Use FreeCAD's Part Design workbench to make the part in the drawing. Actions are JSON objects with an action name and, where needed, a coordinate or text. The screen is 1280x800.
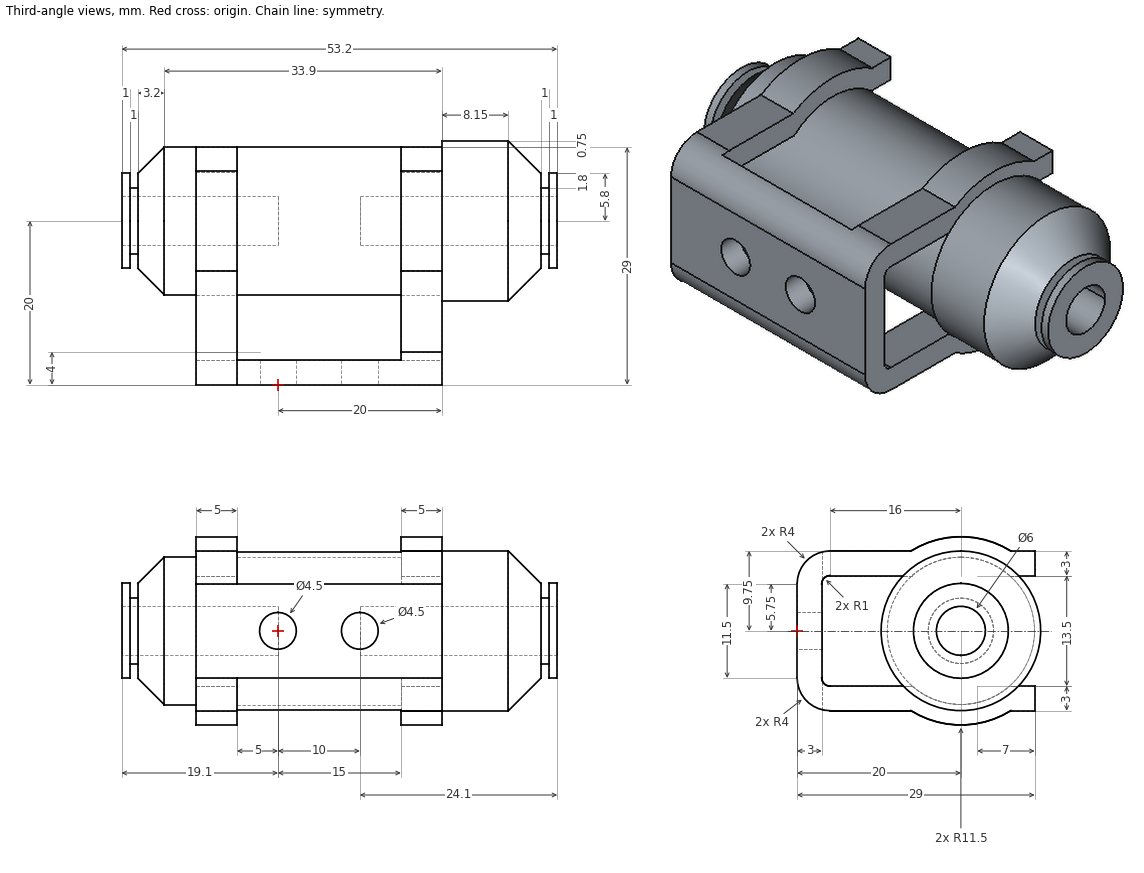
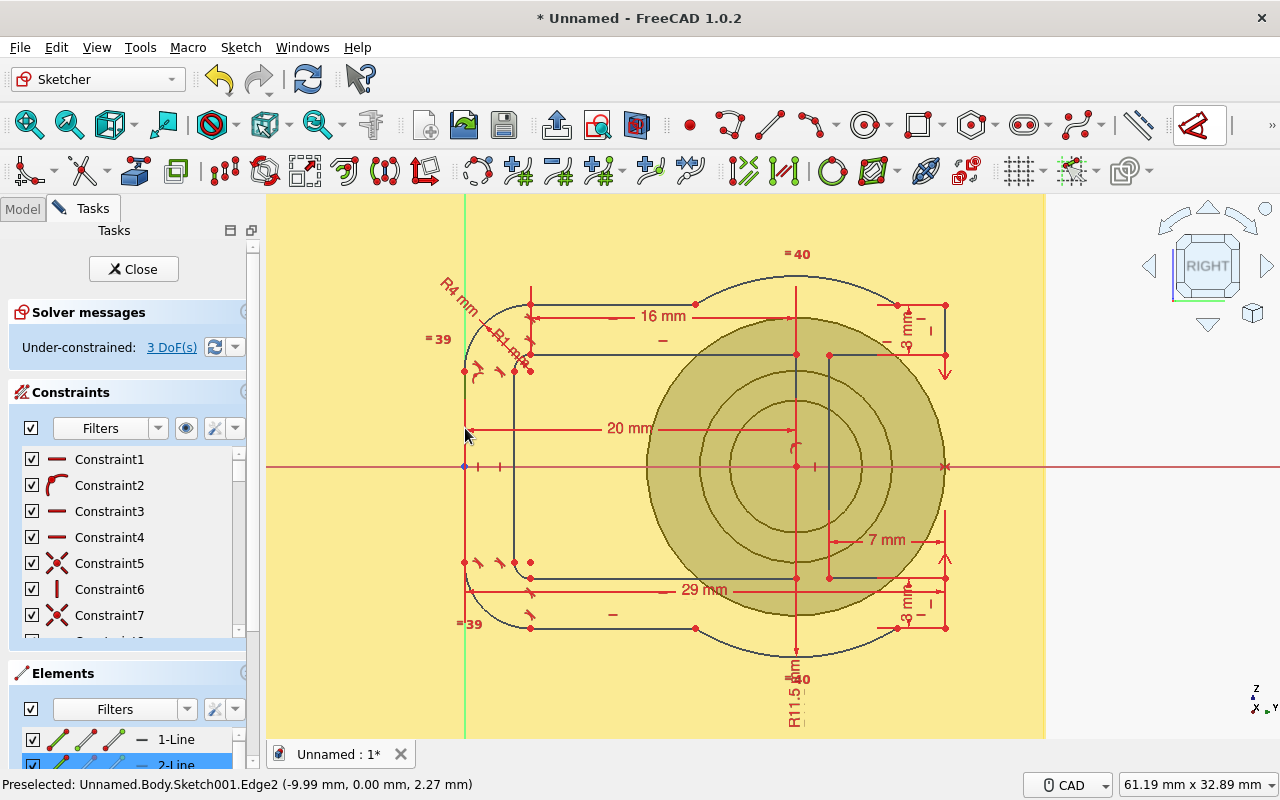
{"action": "left_click", "coordinate": [1220, 126]}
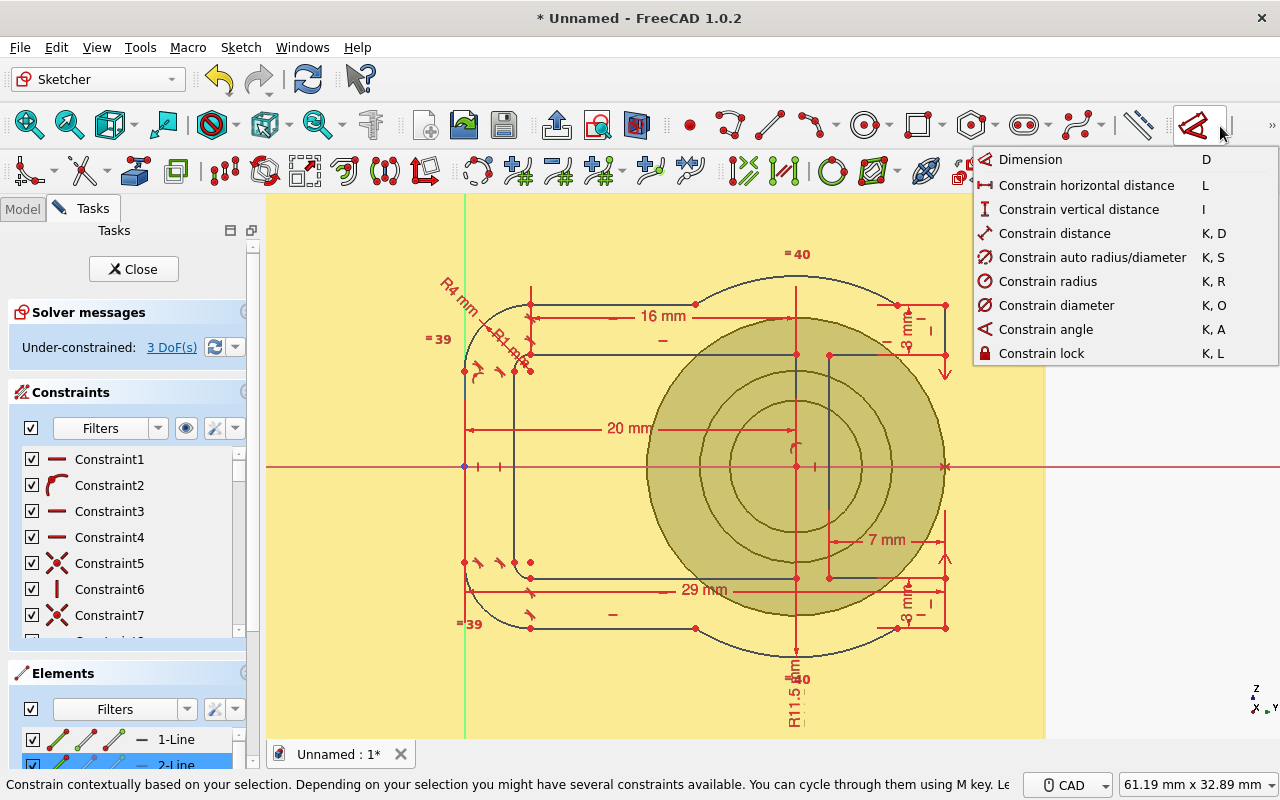
{"action": "left_click", "coordinate": [1126, 209]}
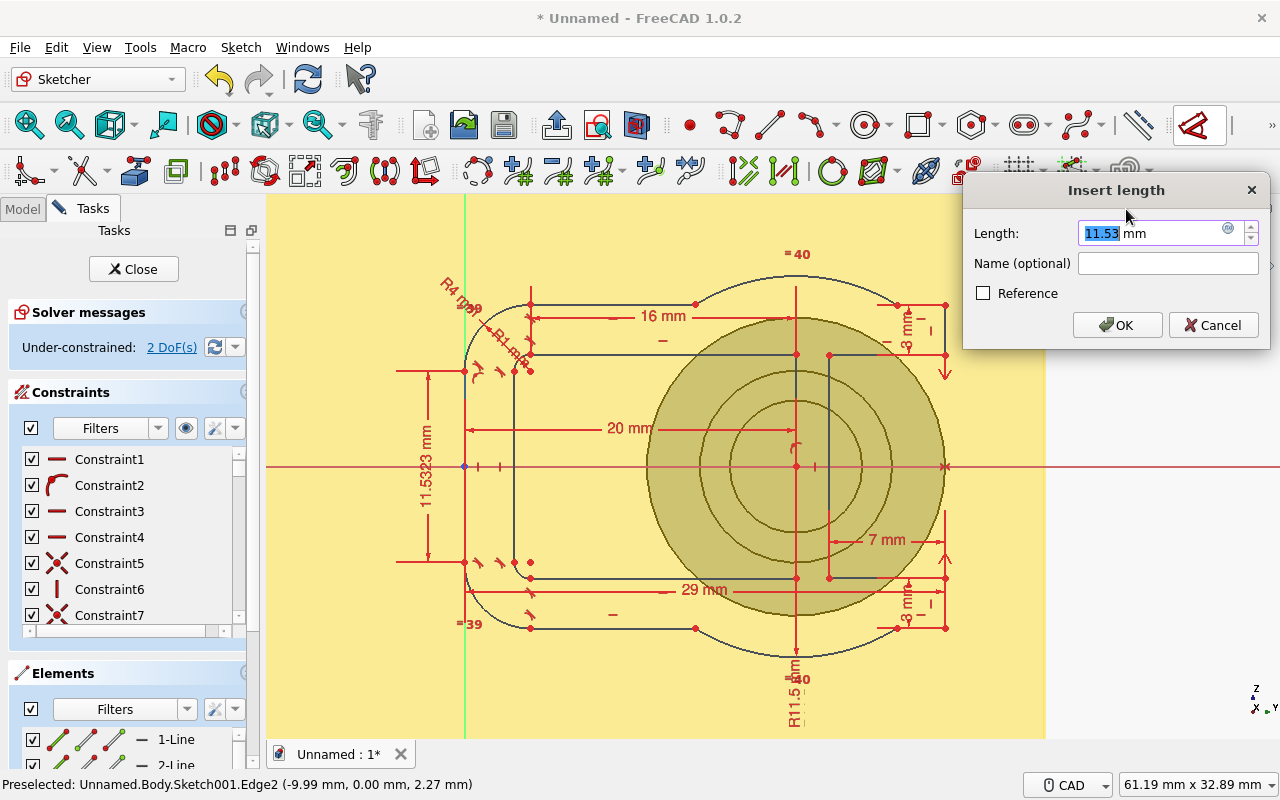
{"action": "type", "text": "11.5"}
{"action": "key", "text": "Return"}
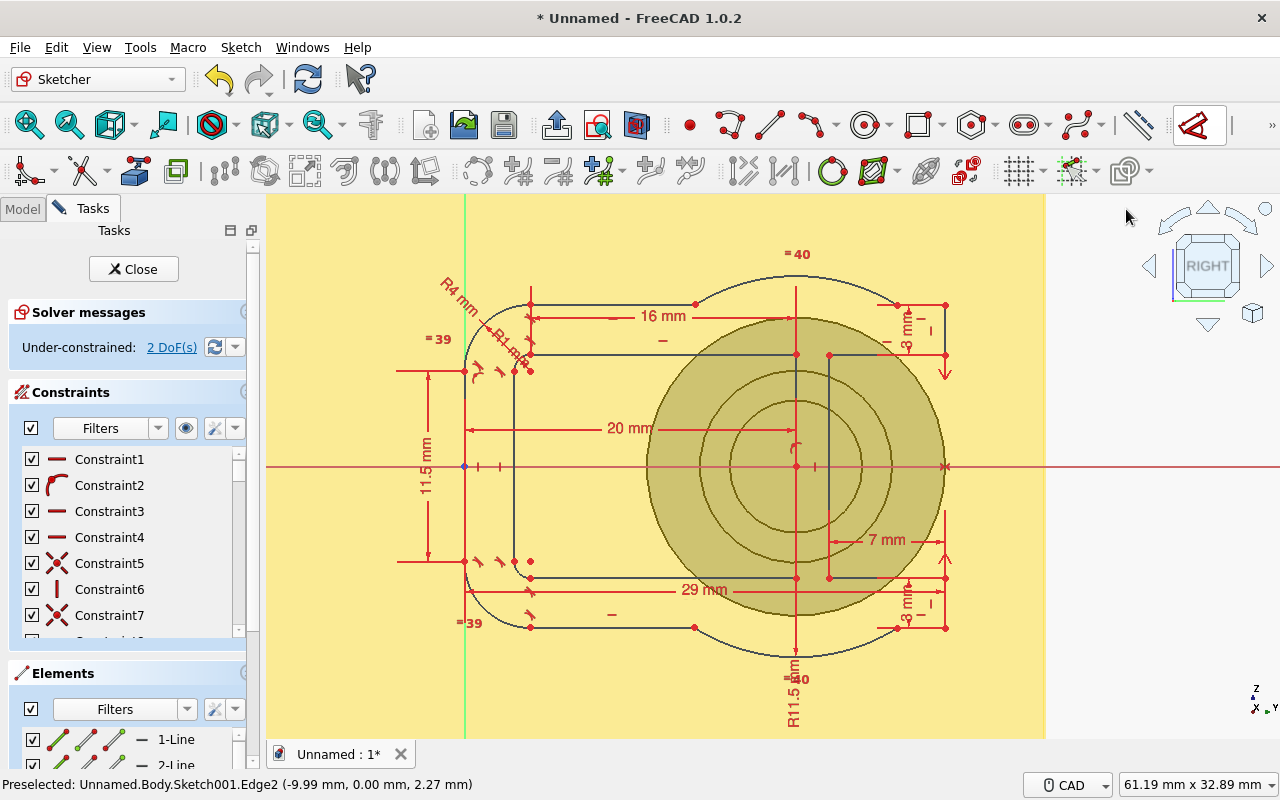
{"action": "left_click", "coordinate": [829, 511]}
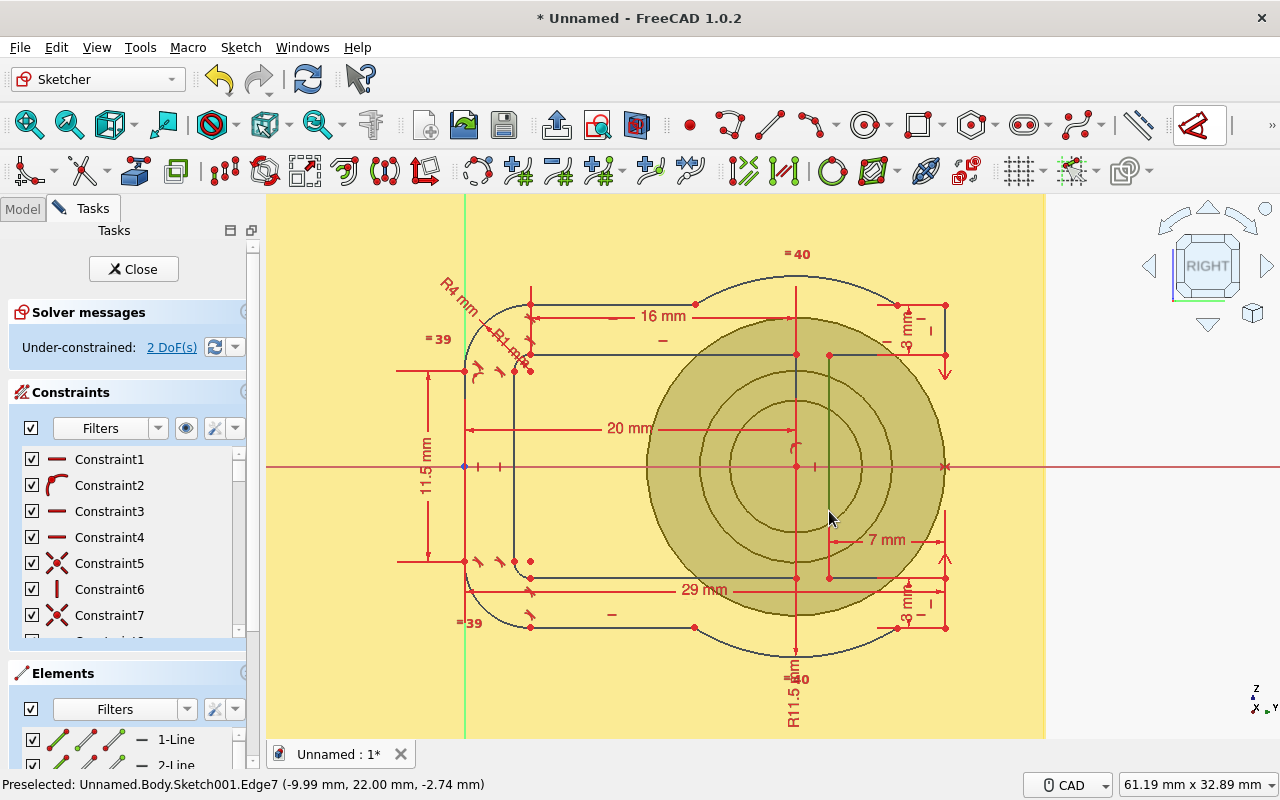
{"action": "key", "text": "i"}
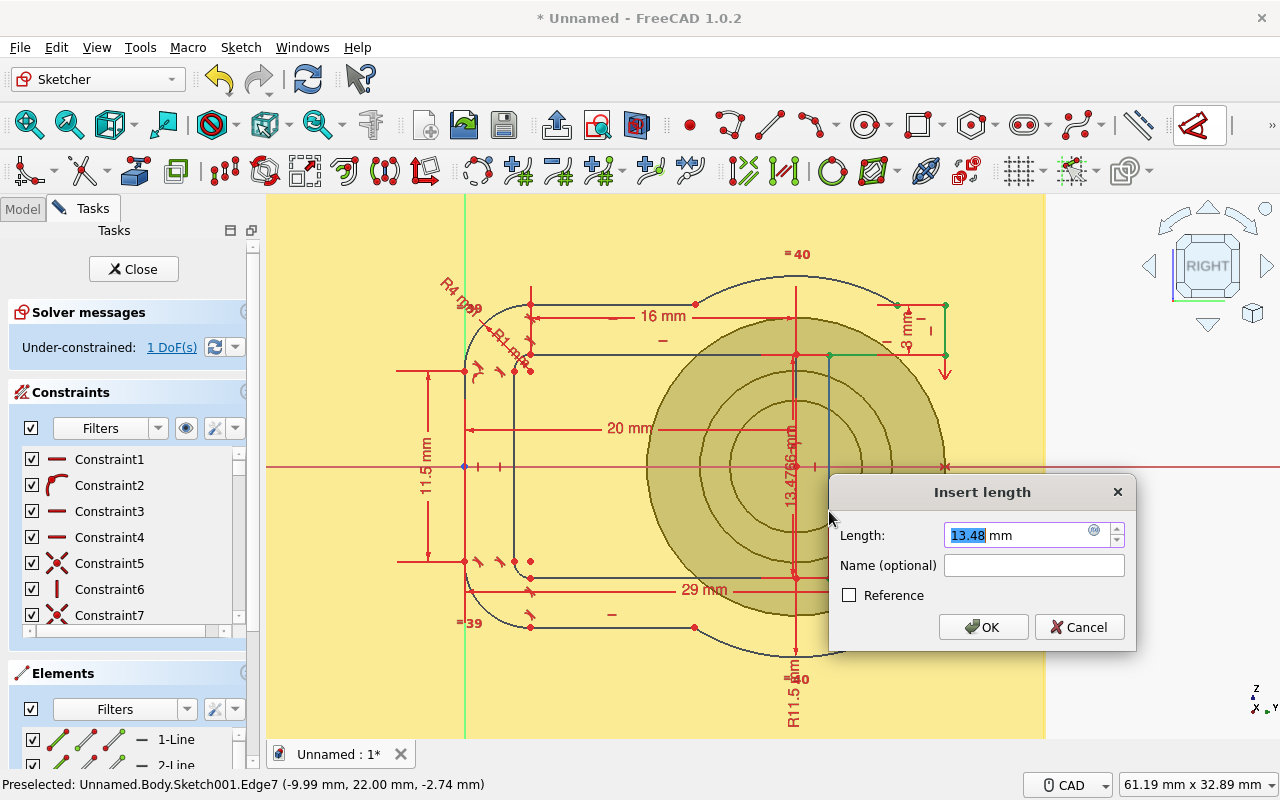
{"action": "type", "text": "13.5"}
{"action": "key", "text": "Return"}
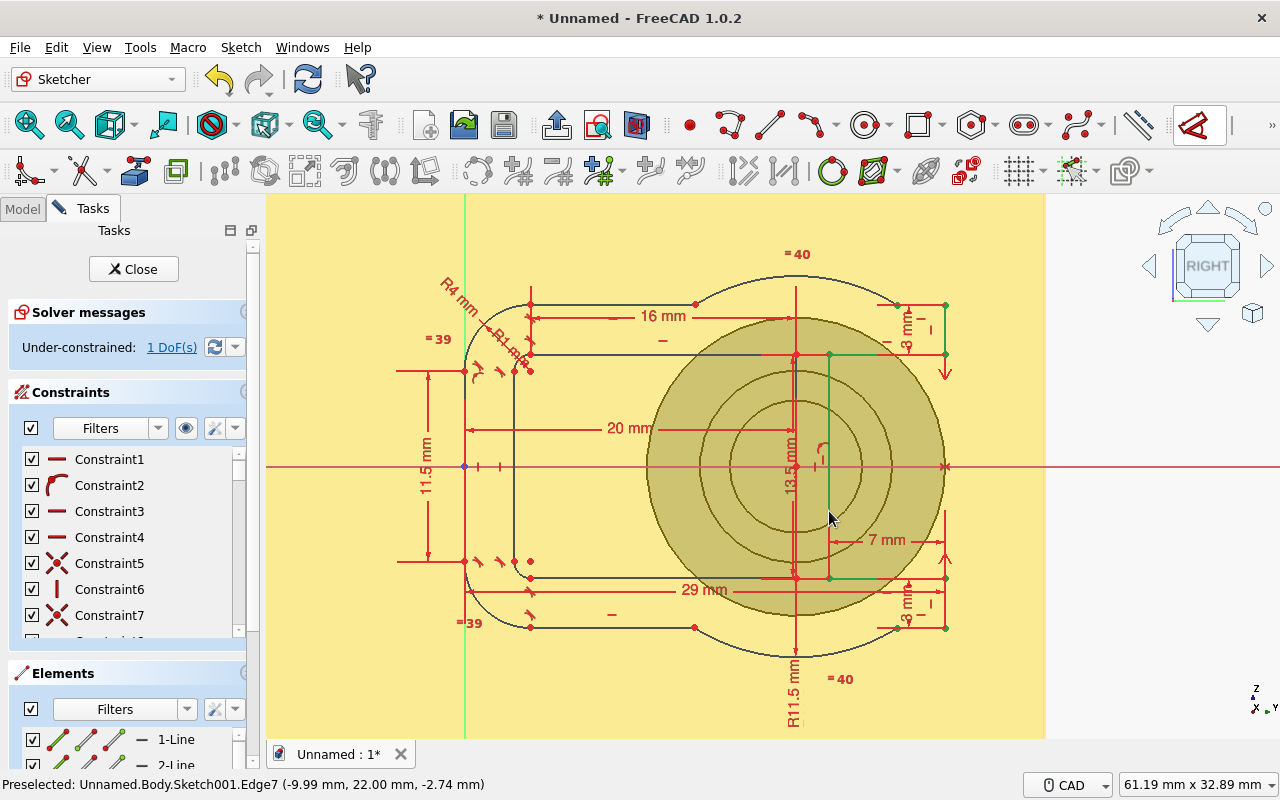
{"action": "left_click", "coordinate": [695, 305]}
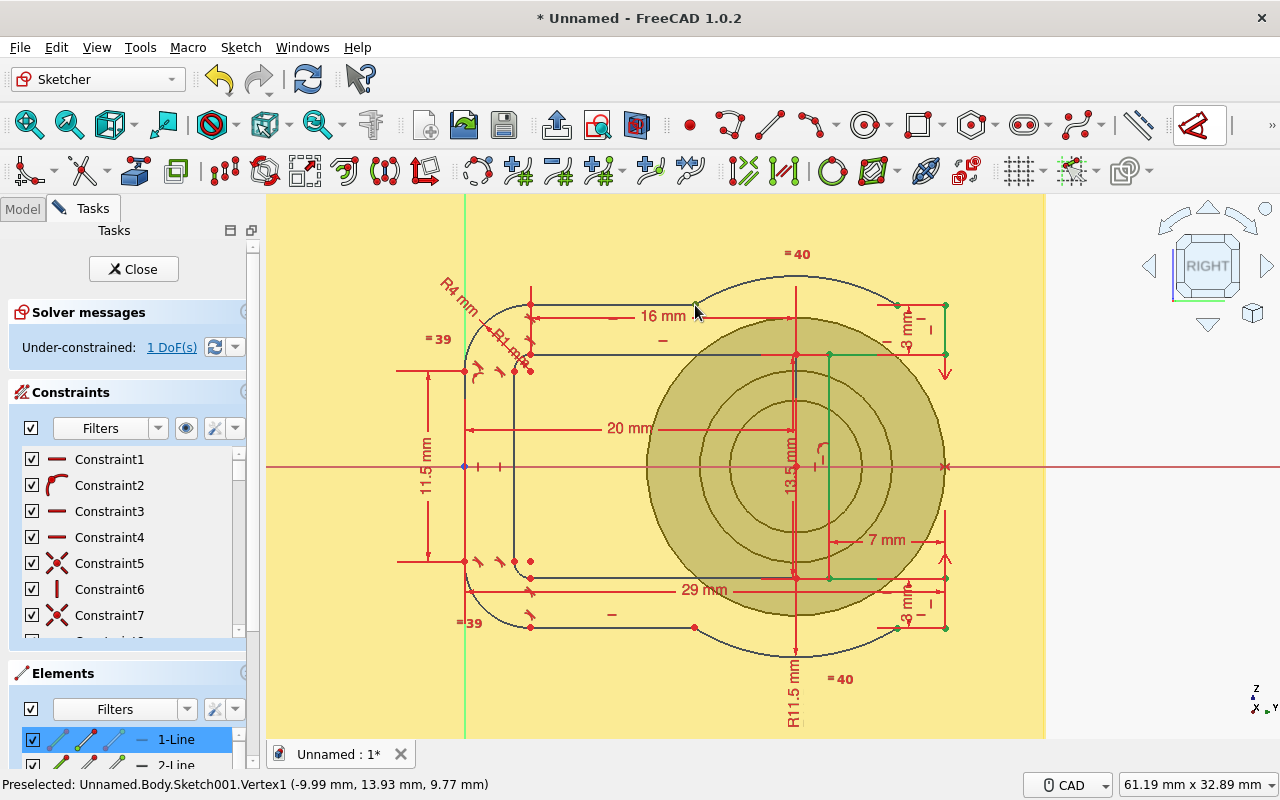
{"action": "key", "text": "i"}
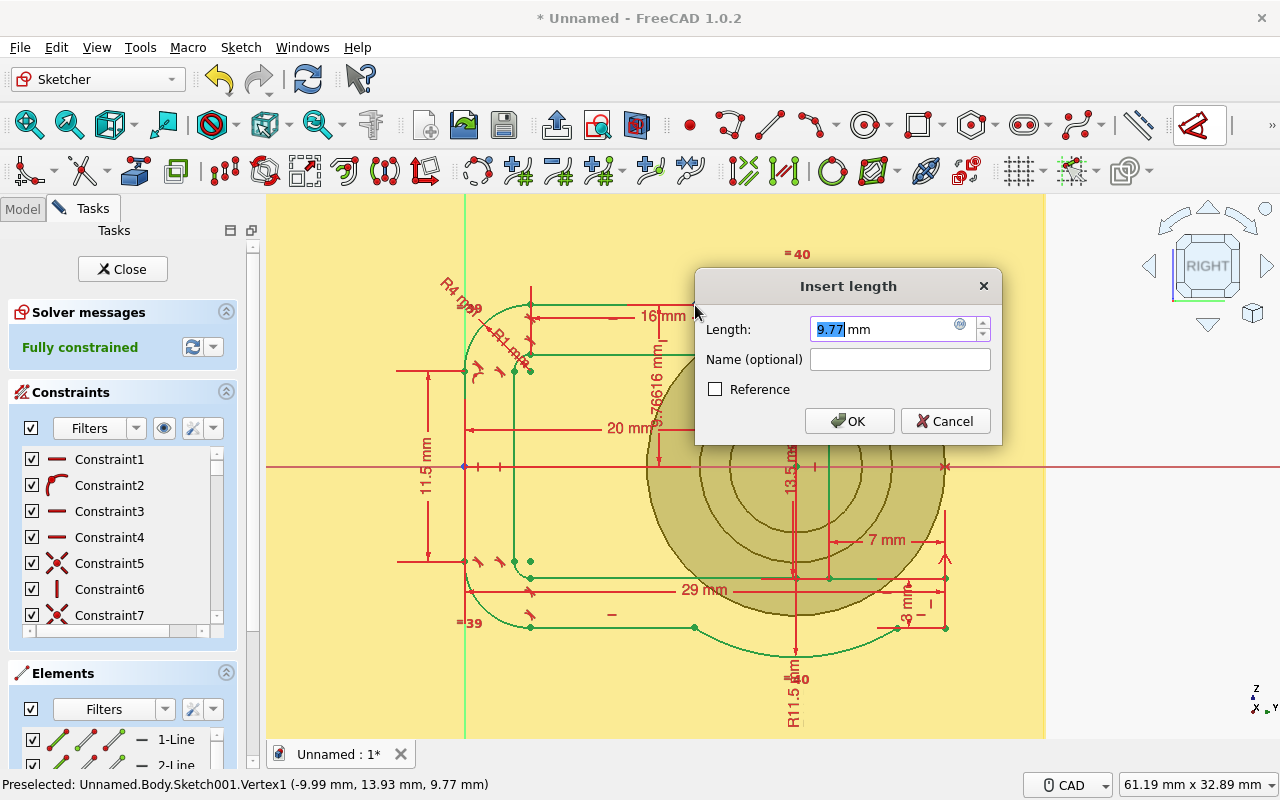
{"action": "type", "text": "9.75"}
{"action": "key", "text": "Return"}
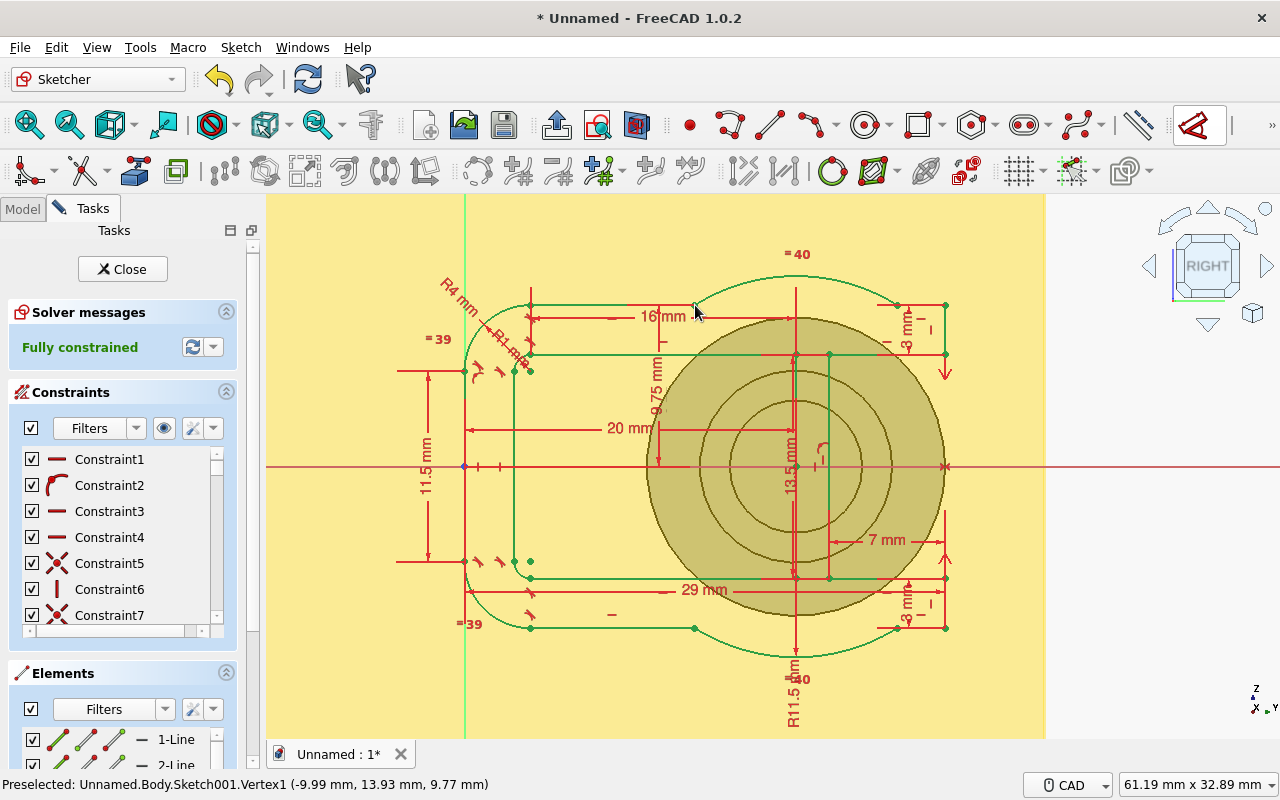
{"action": "left_click", "coordinate": [123, 269]}